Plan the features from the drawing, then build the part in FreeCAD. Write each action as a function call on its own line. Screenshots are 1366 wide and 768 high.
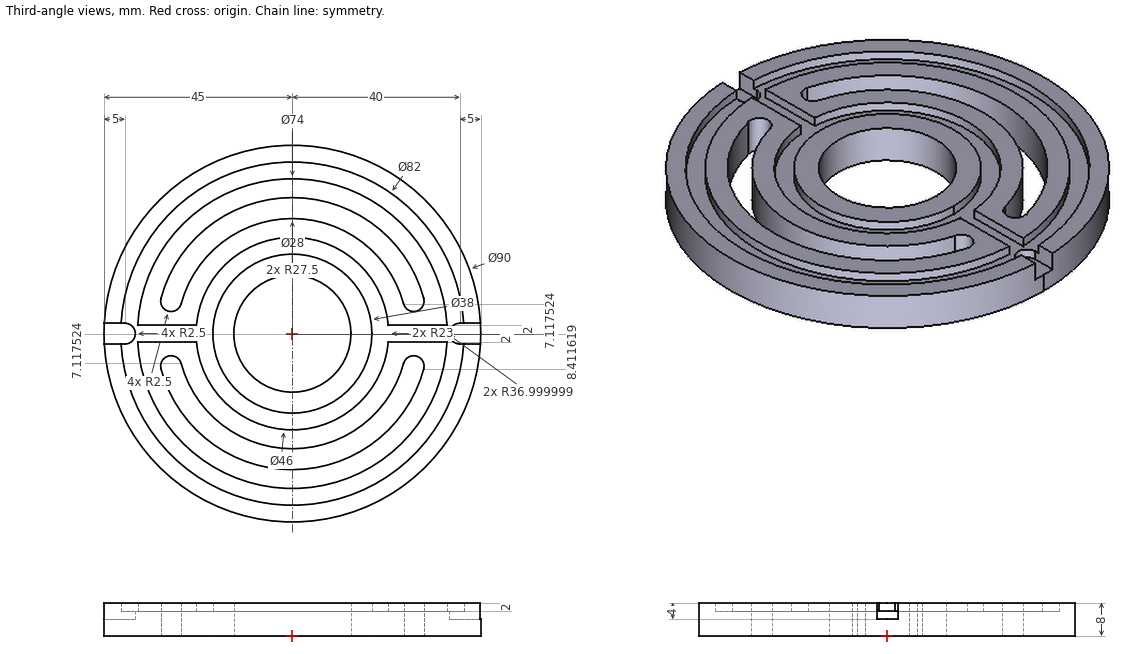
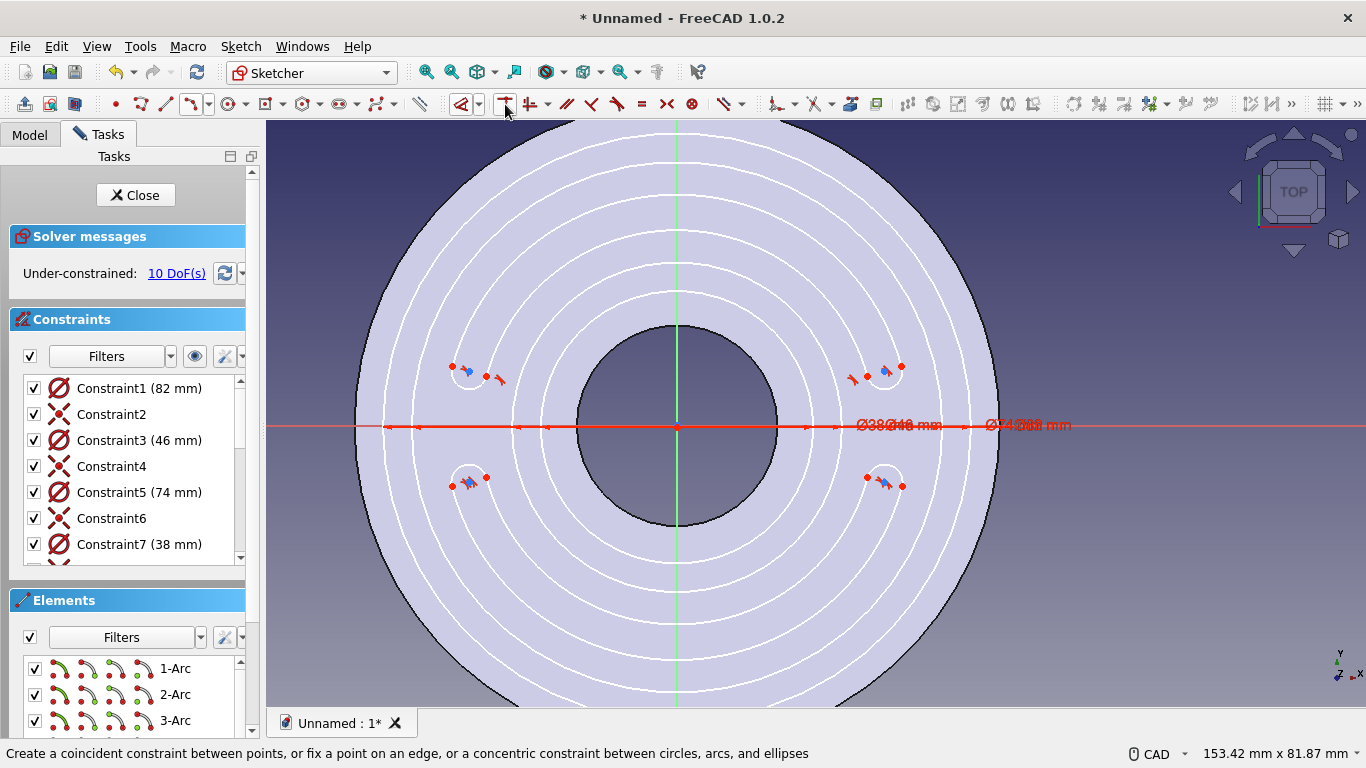
scroll(677, 427, up, 5)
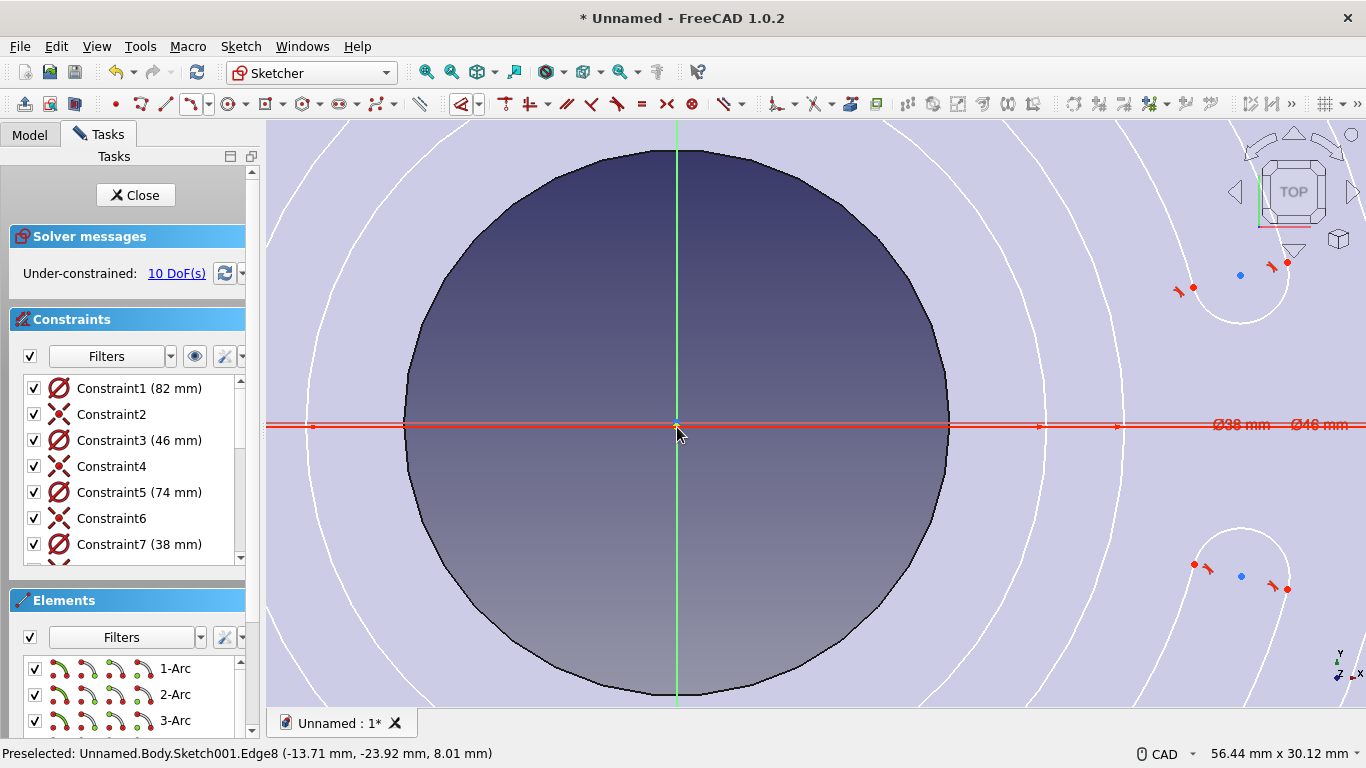
drag(666, 413, 687, 437)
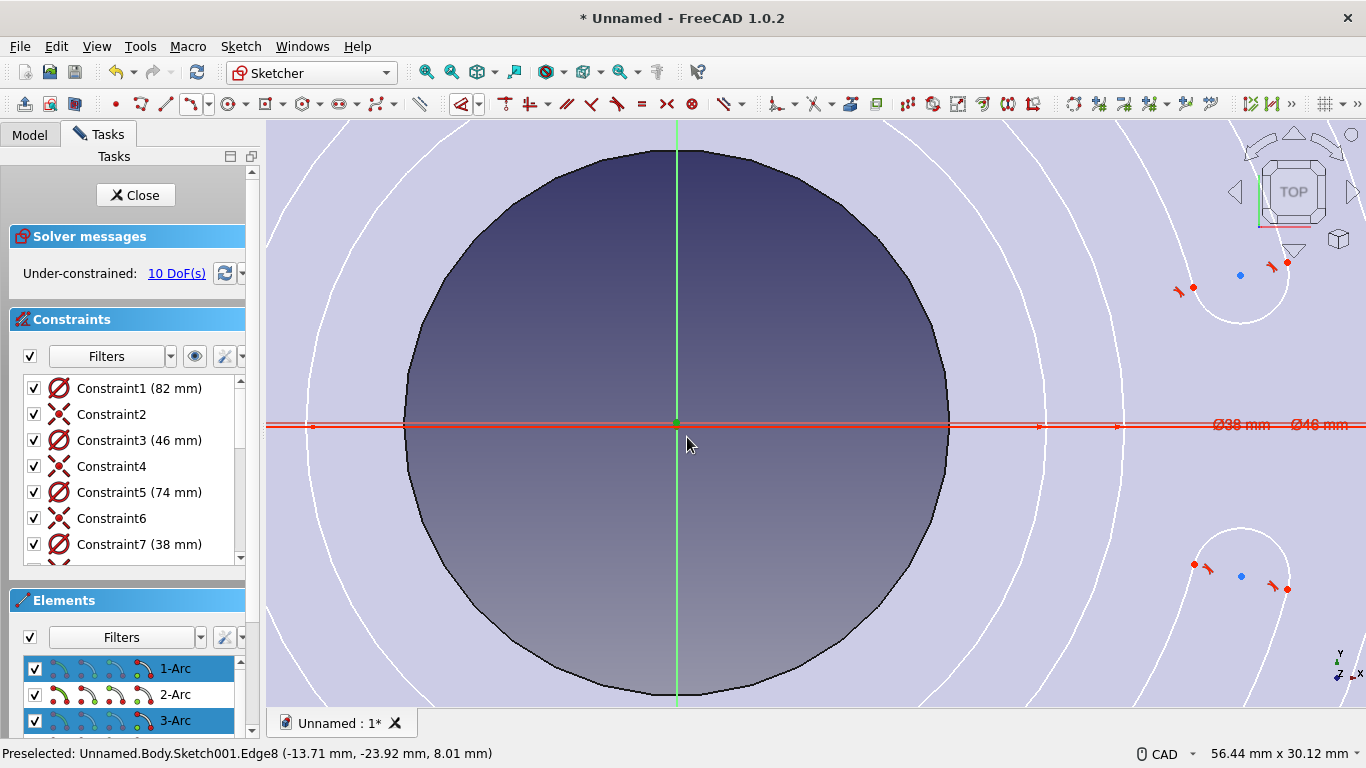
key(c)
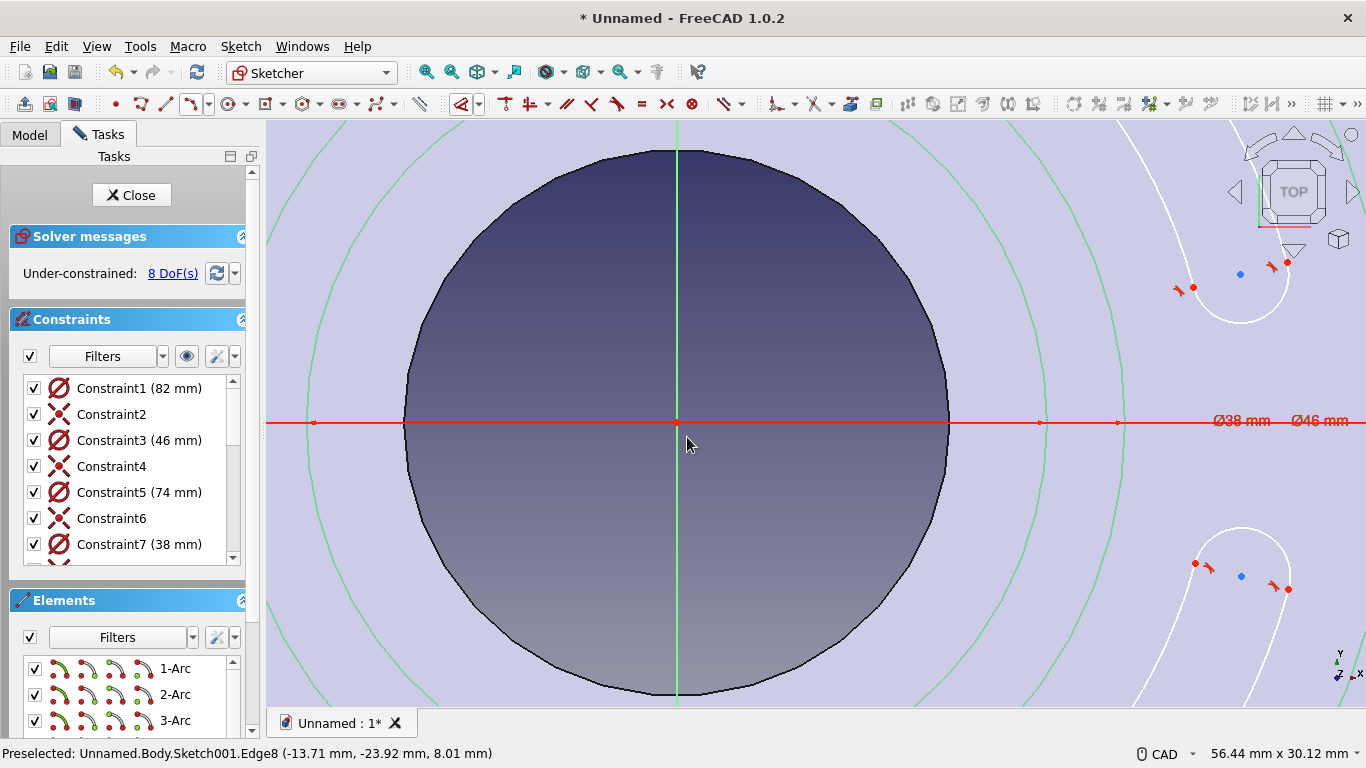
scroll(771, 410, down, 7)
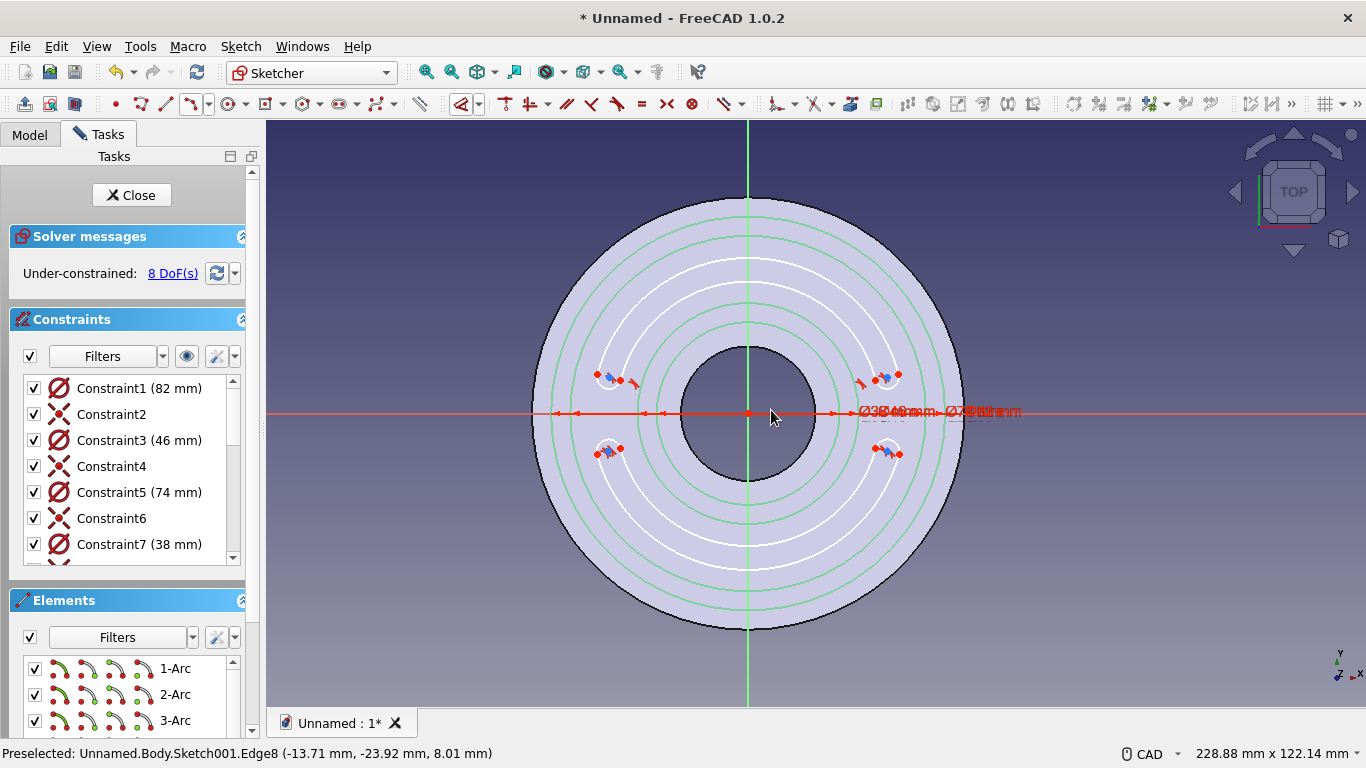
scroll(883, 388, up, 2)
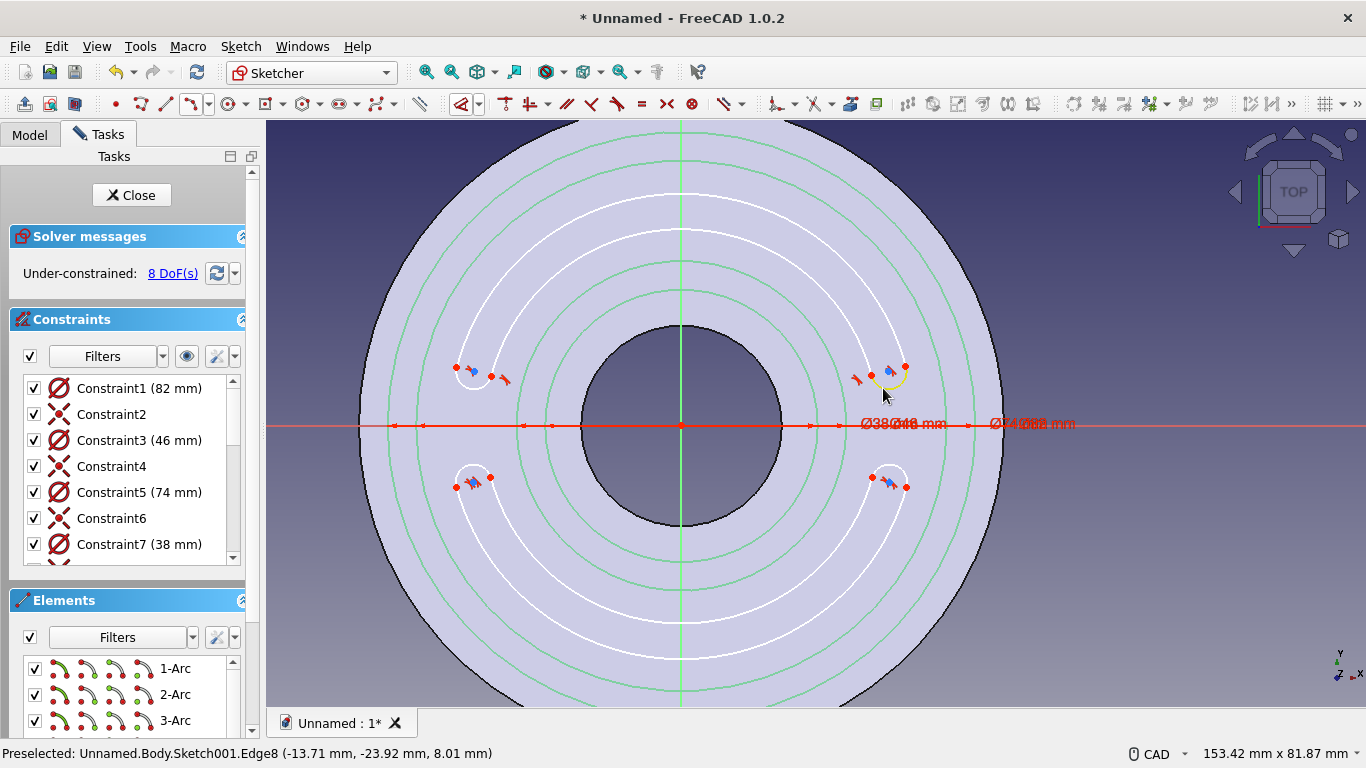
click(882, 388)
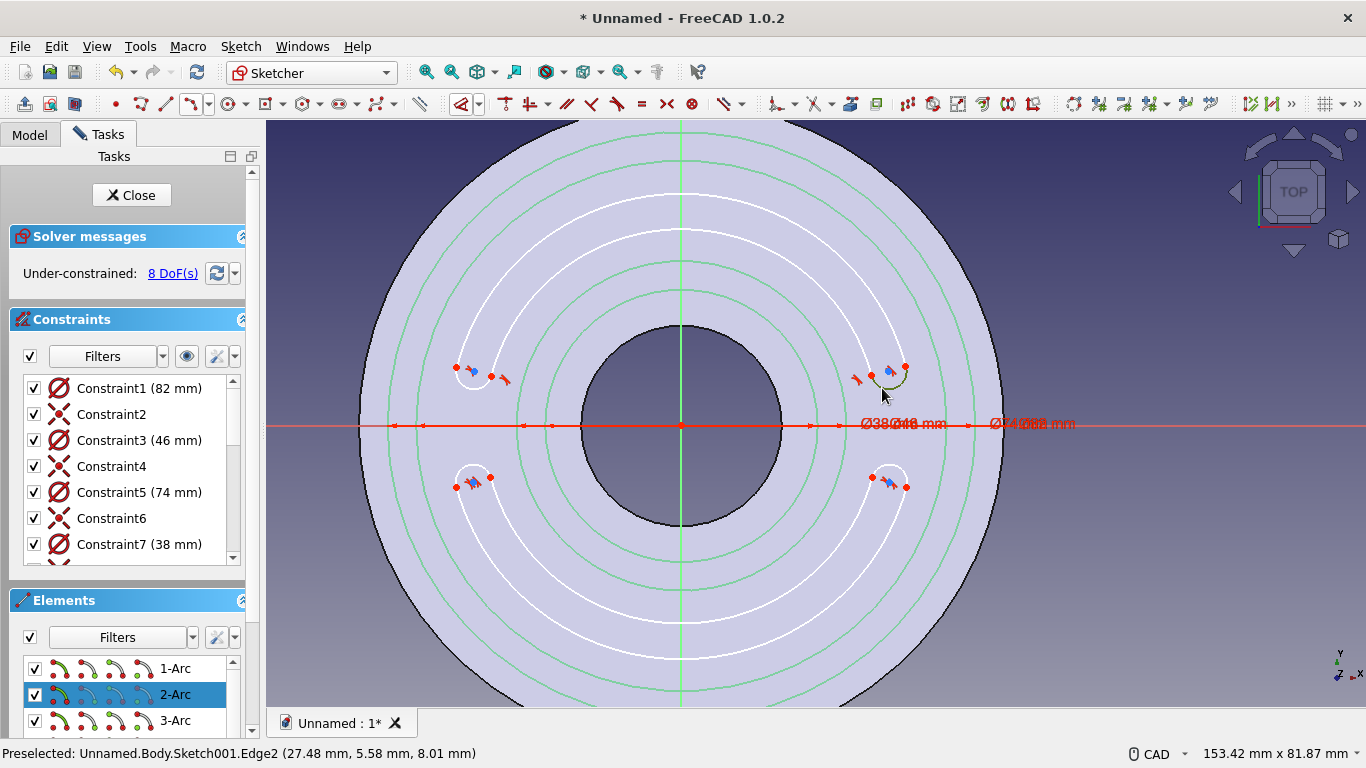
click(480, 466)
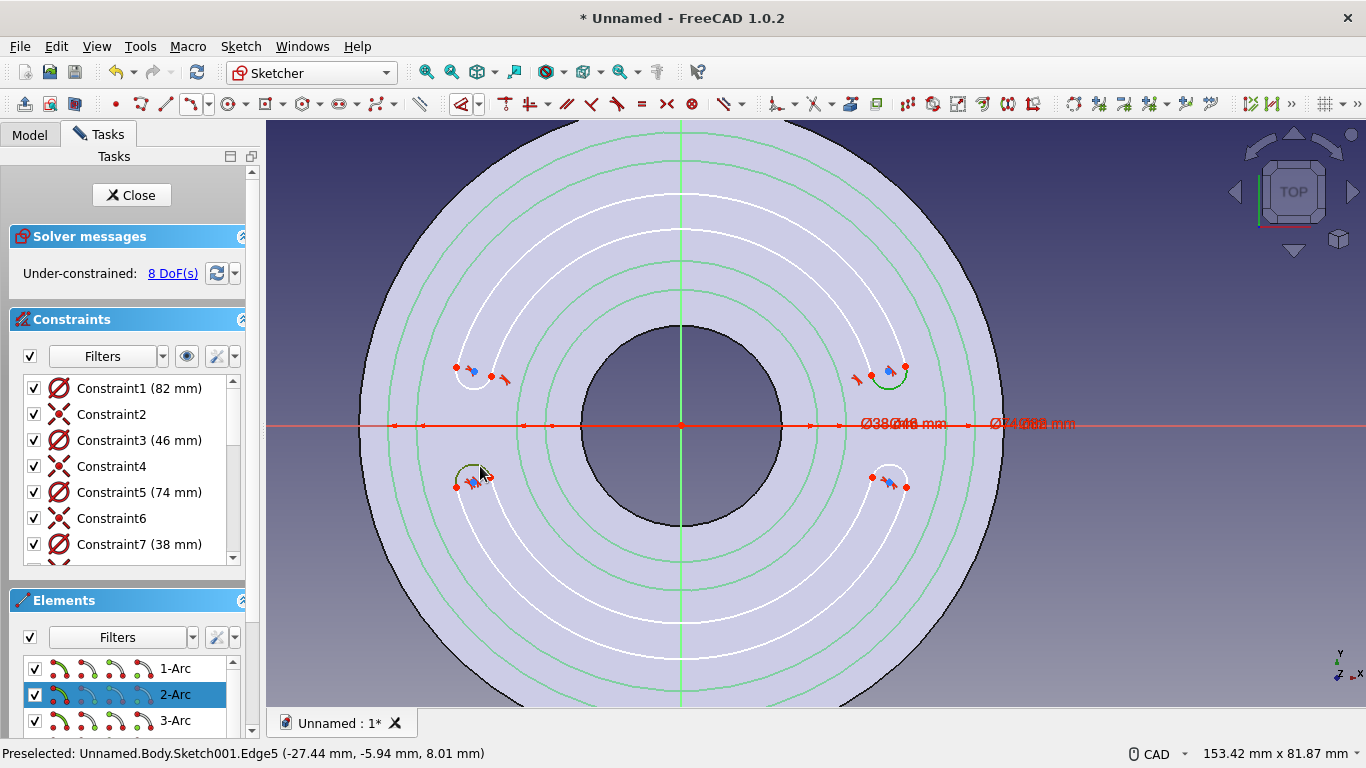
key(e)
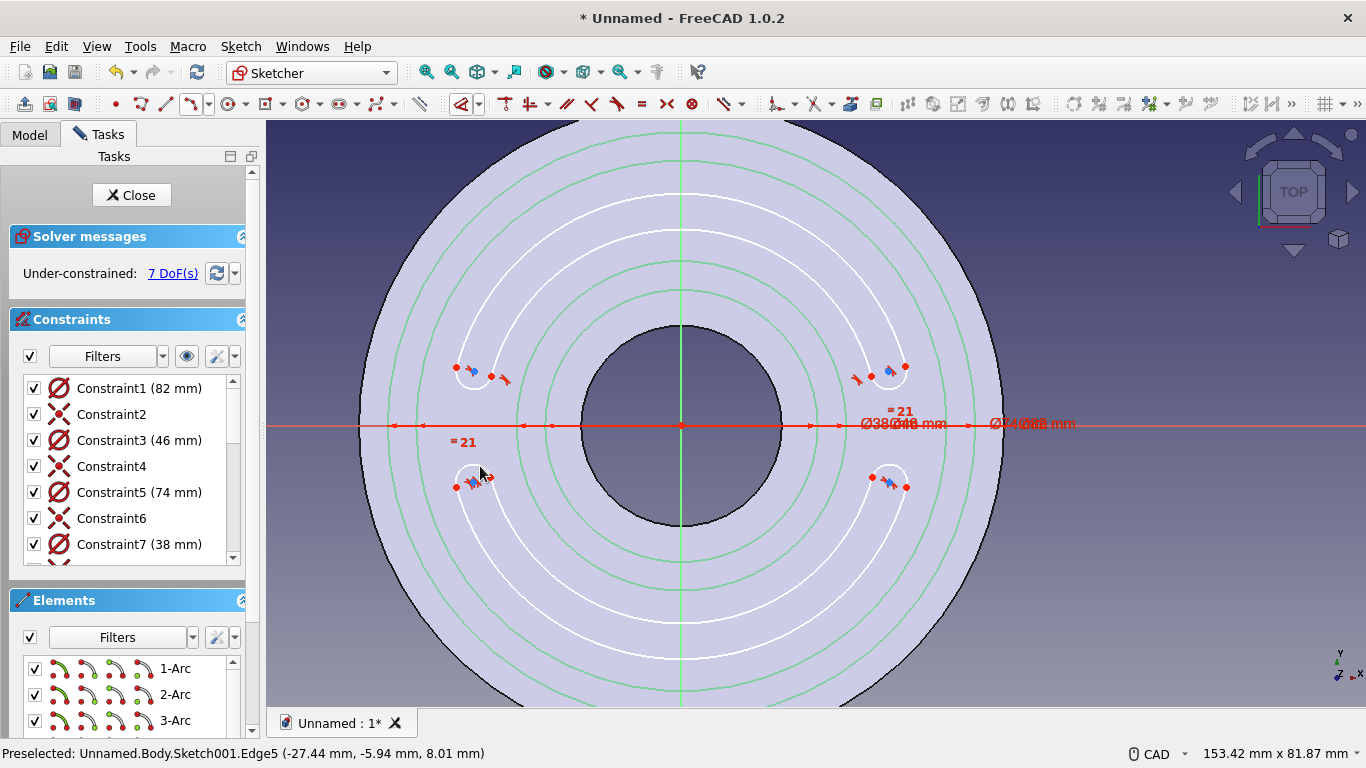
click(798, 225)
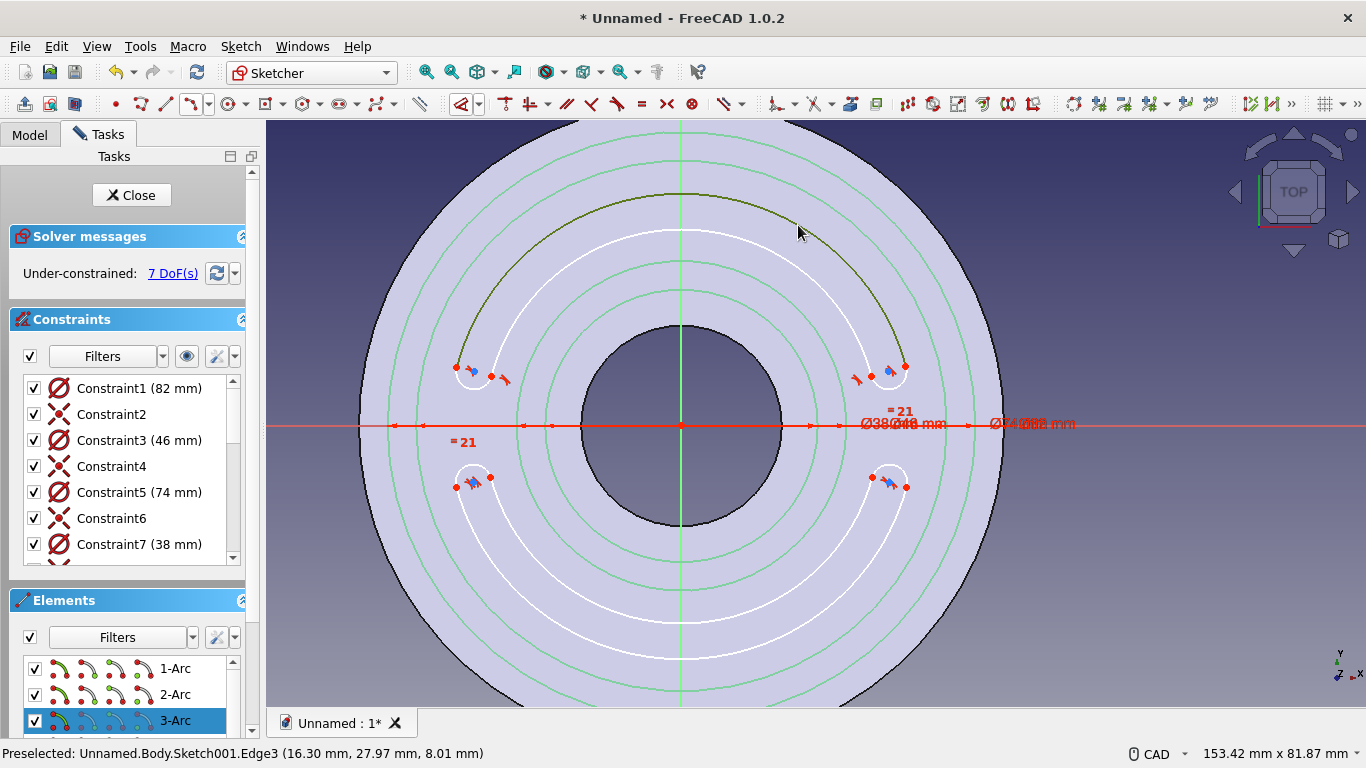
click(565, 628)